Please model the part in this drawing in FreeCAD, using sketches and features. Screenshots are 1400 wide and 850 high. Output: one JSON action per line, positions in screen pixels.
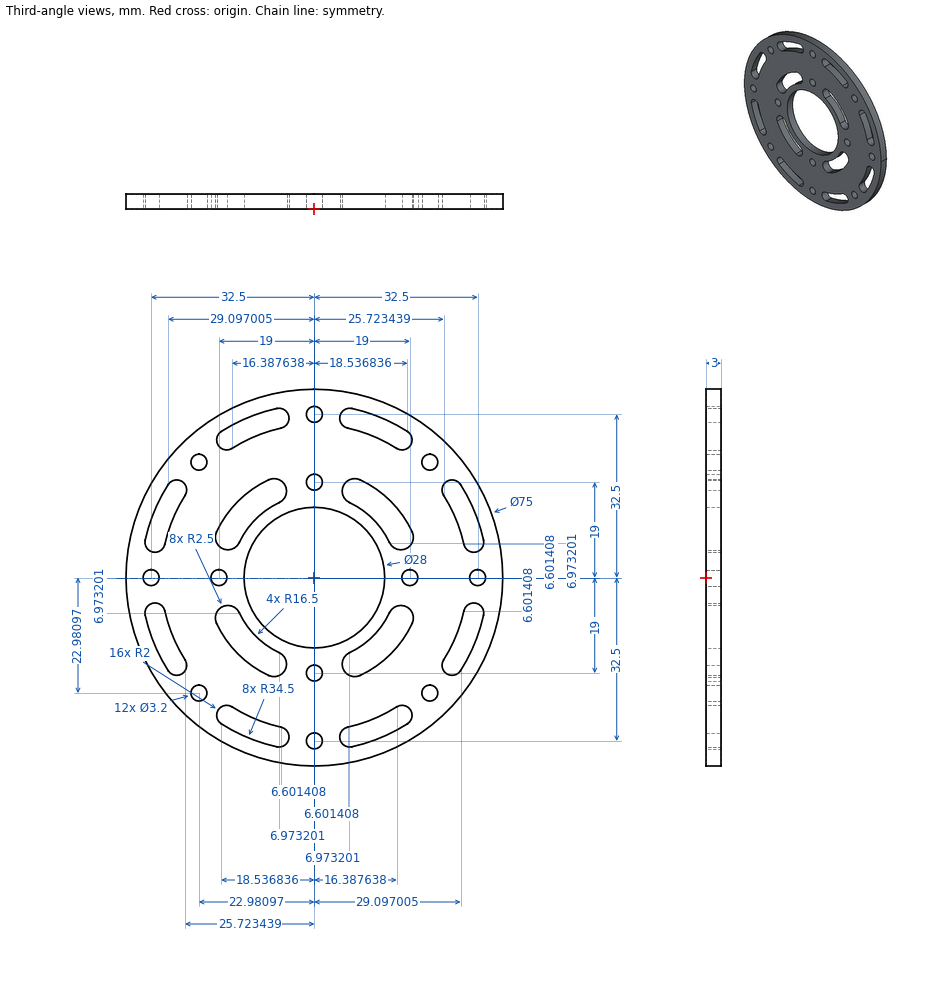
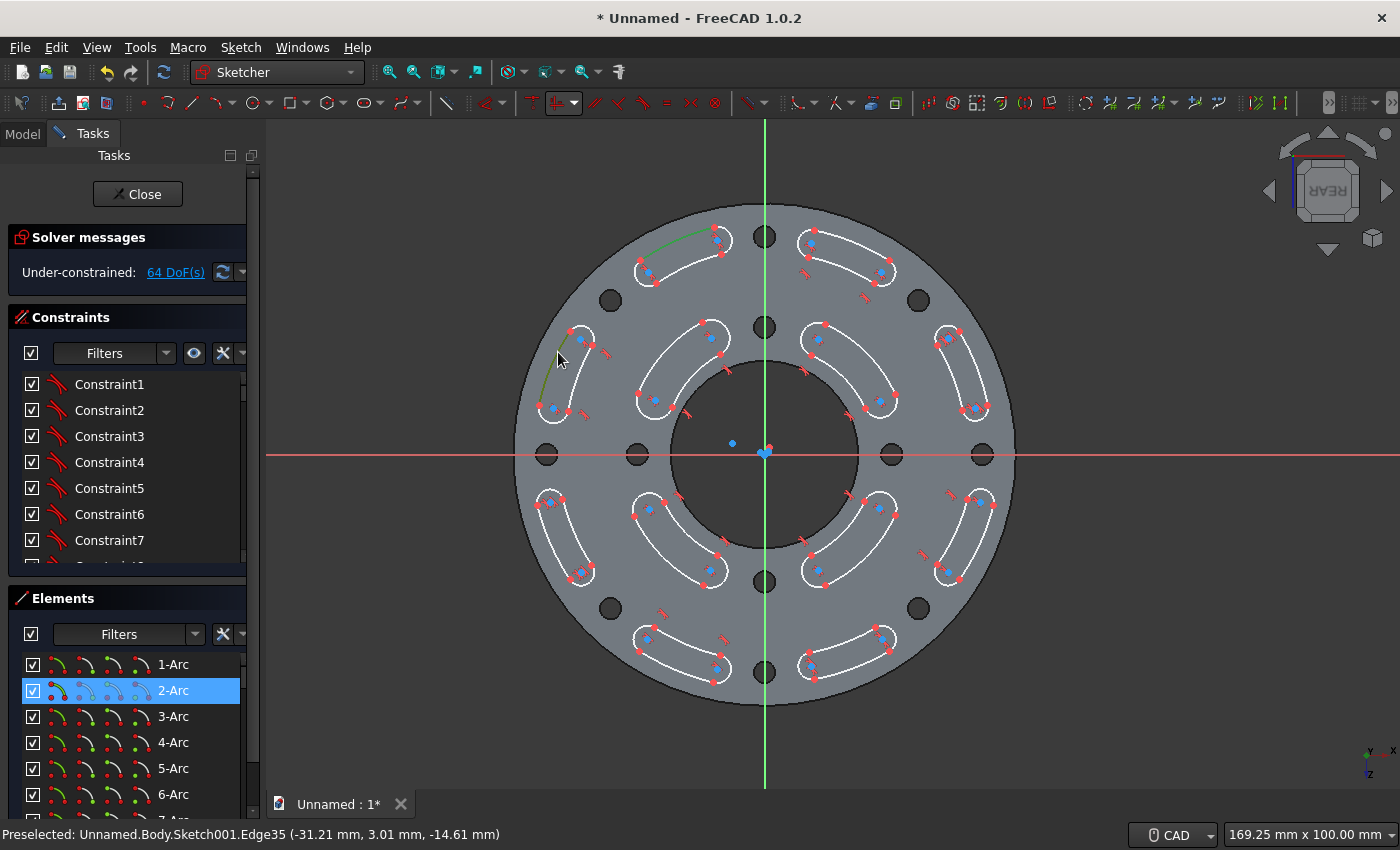
{"action": "left_click", "coordinate": [532, 104]}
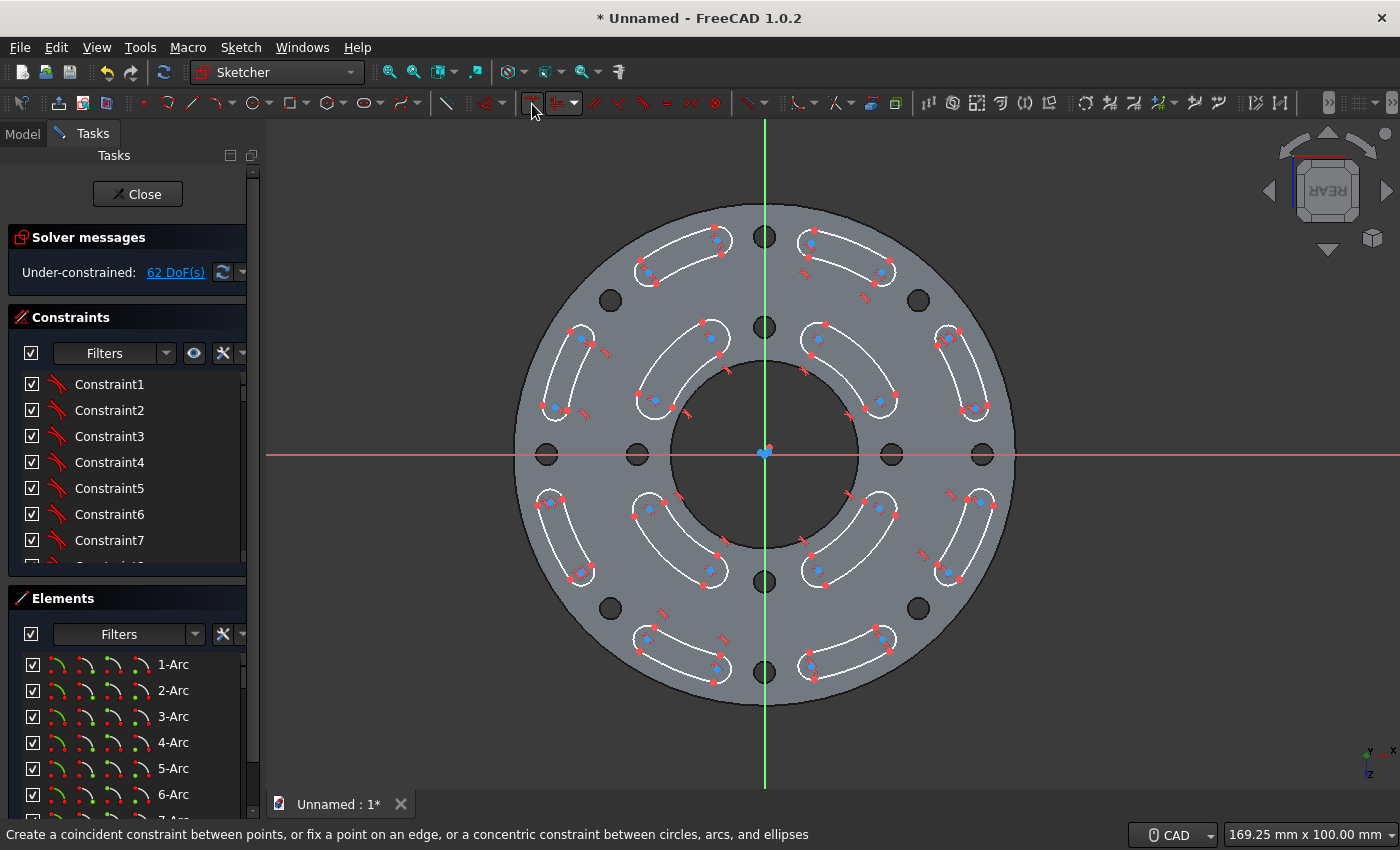
{"action": "left_click", "coordinate": [691, 234]}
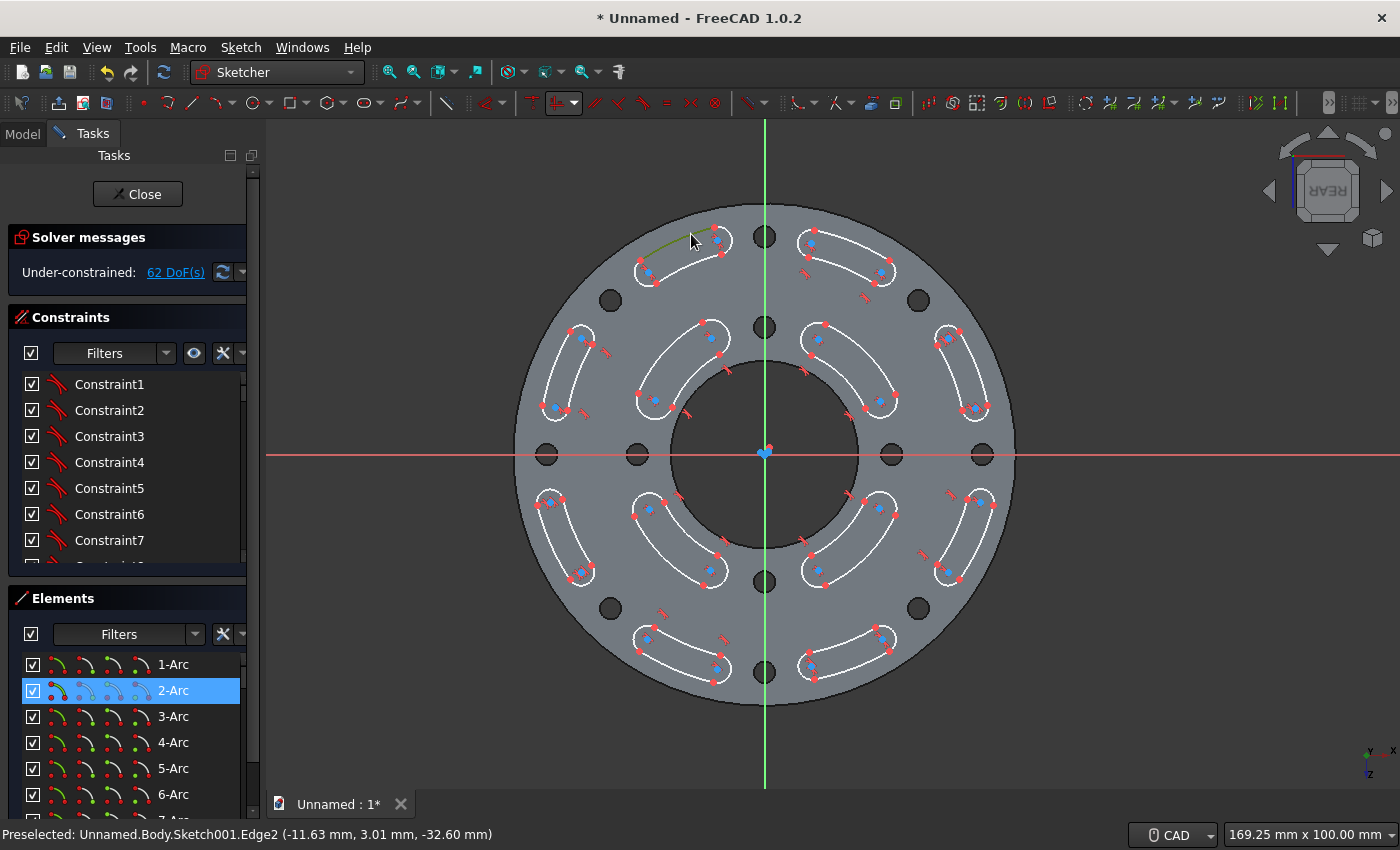
{"action": "left_click", "coordinate": [853, 388]}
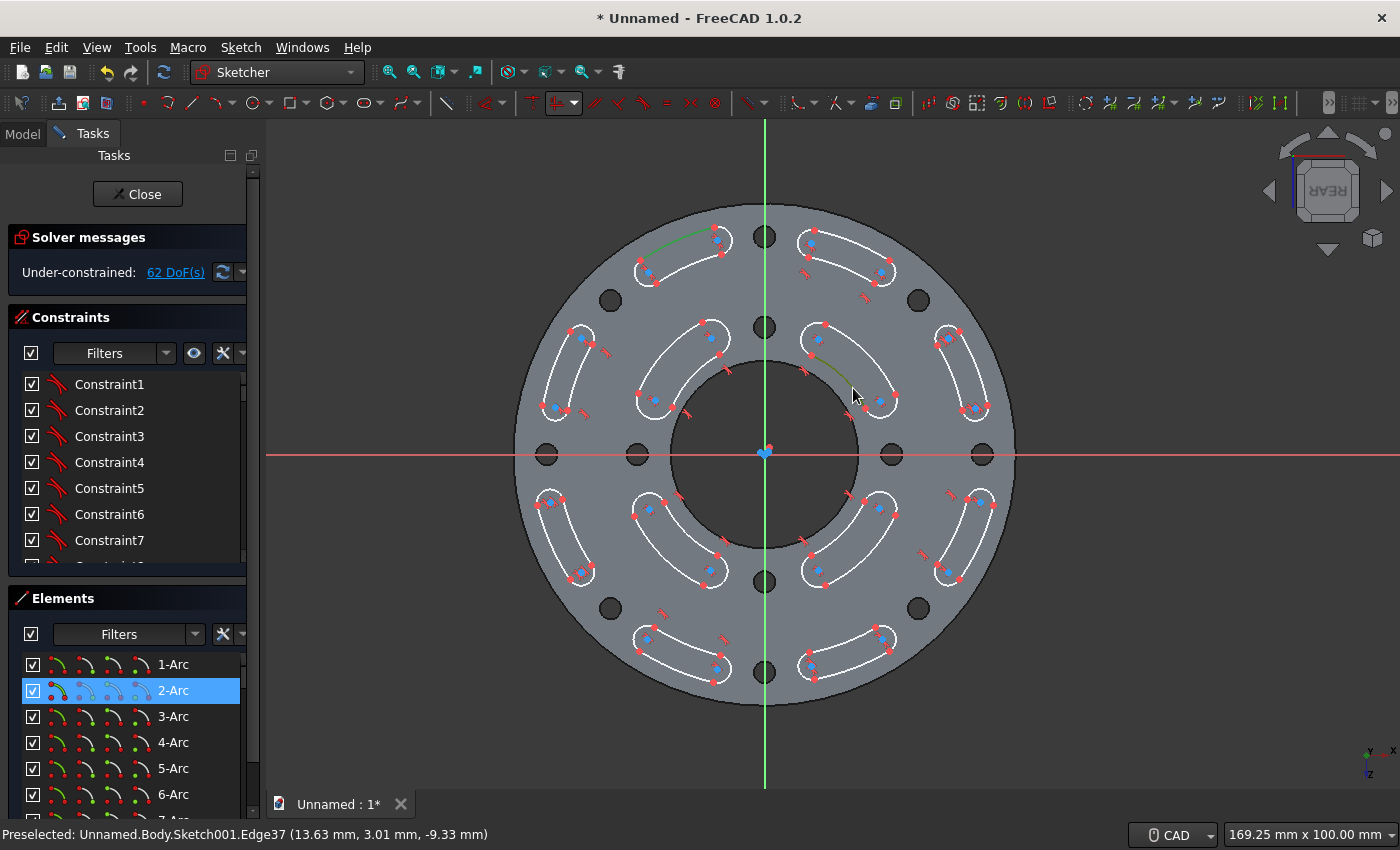
{"action": "left_click", "coordinate": [532, 104]}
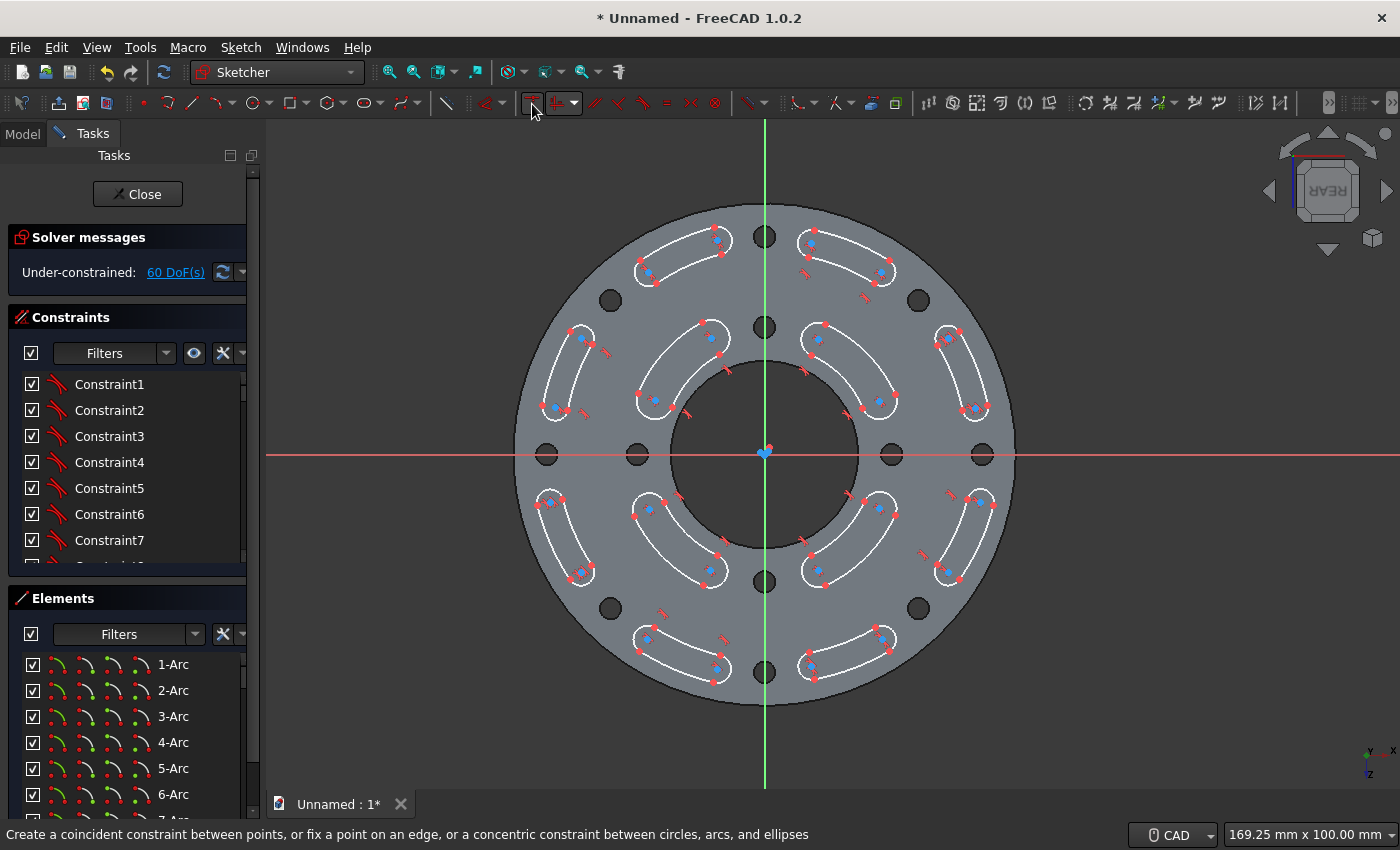
{"action": "left_click", "coordinate": [691, 235]}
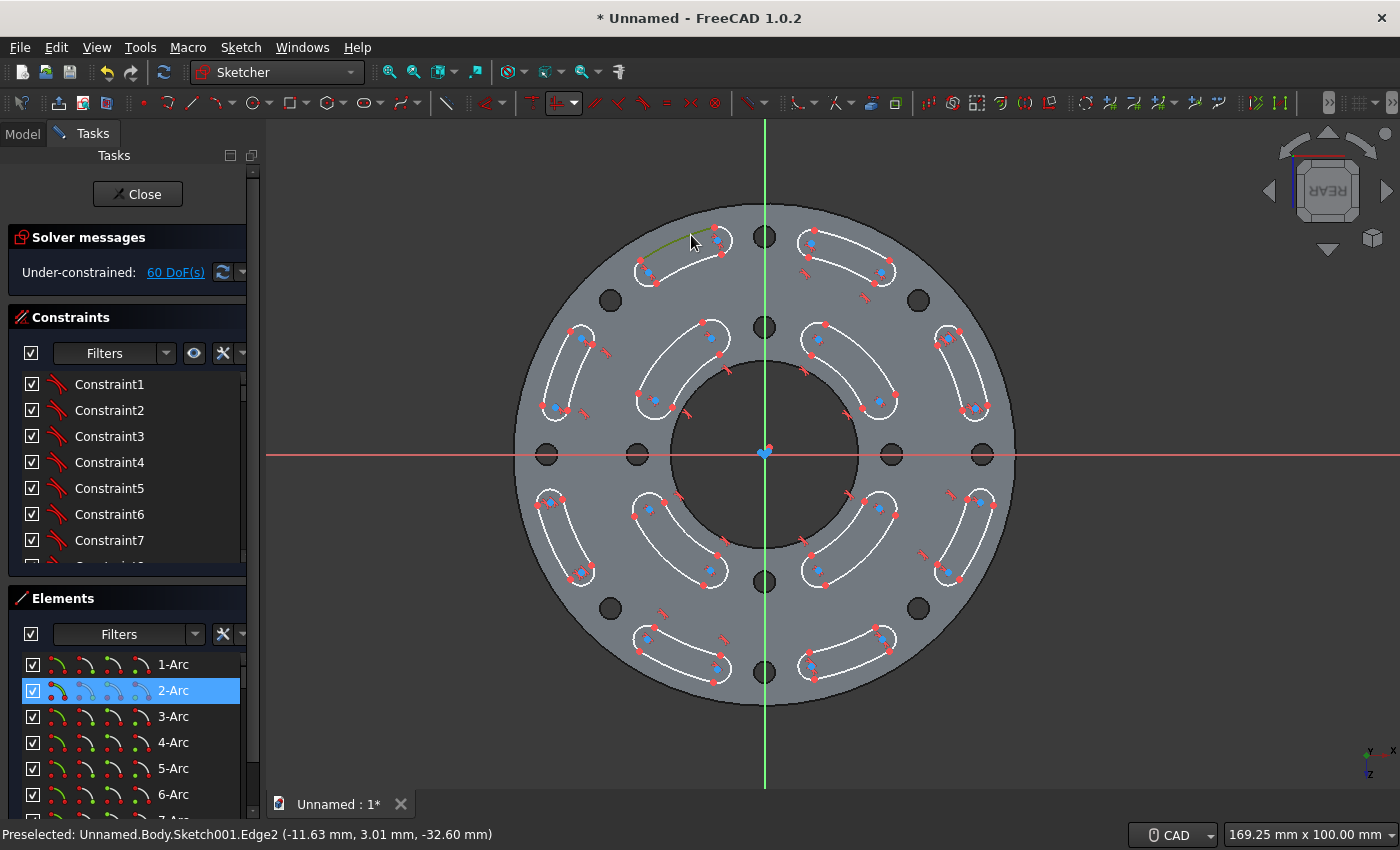
{"action": "left_click", "coordinate": [880, 368]}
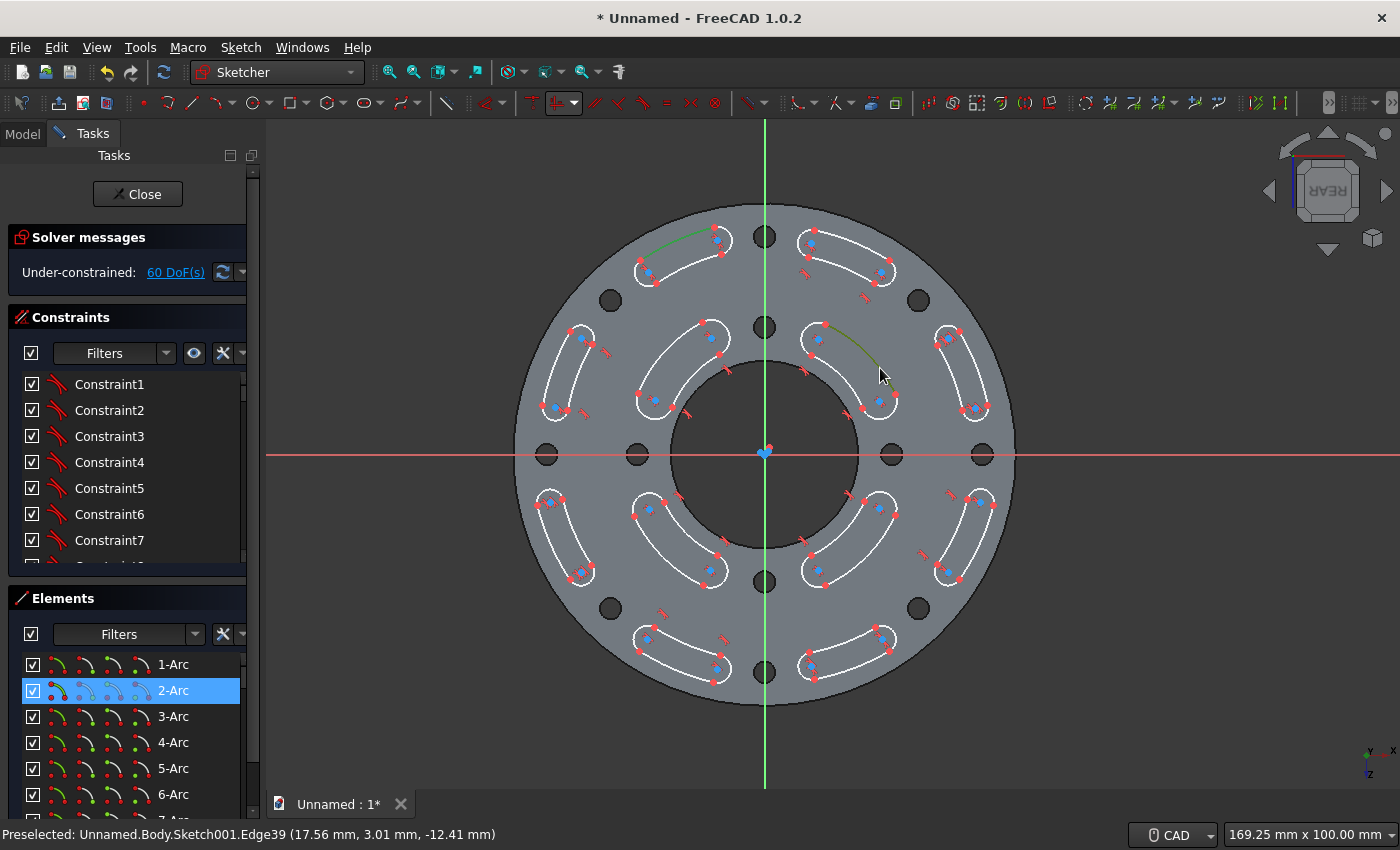
{"action": "left_click", "coordinate": [532, 104]}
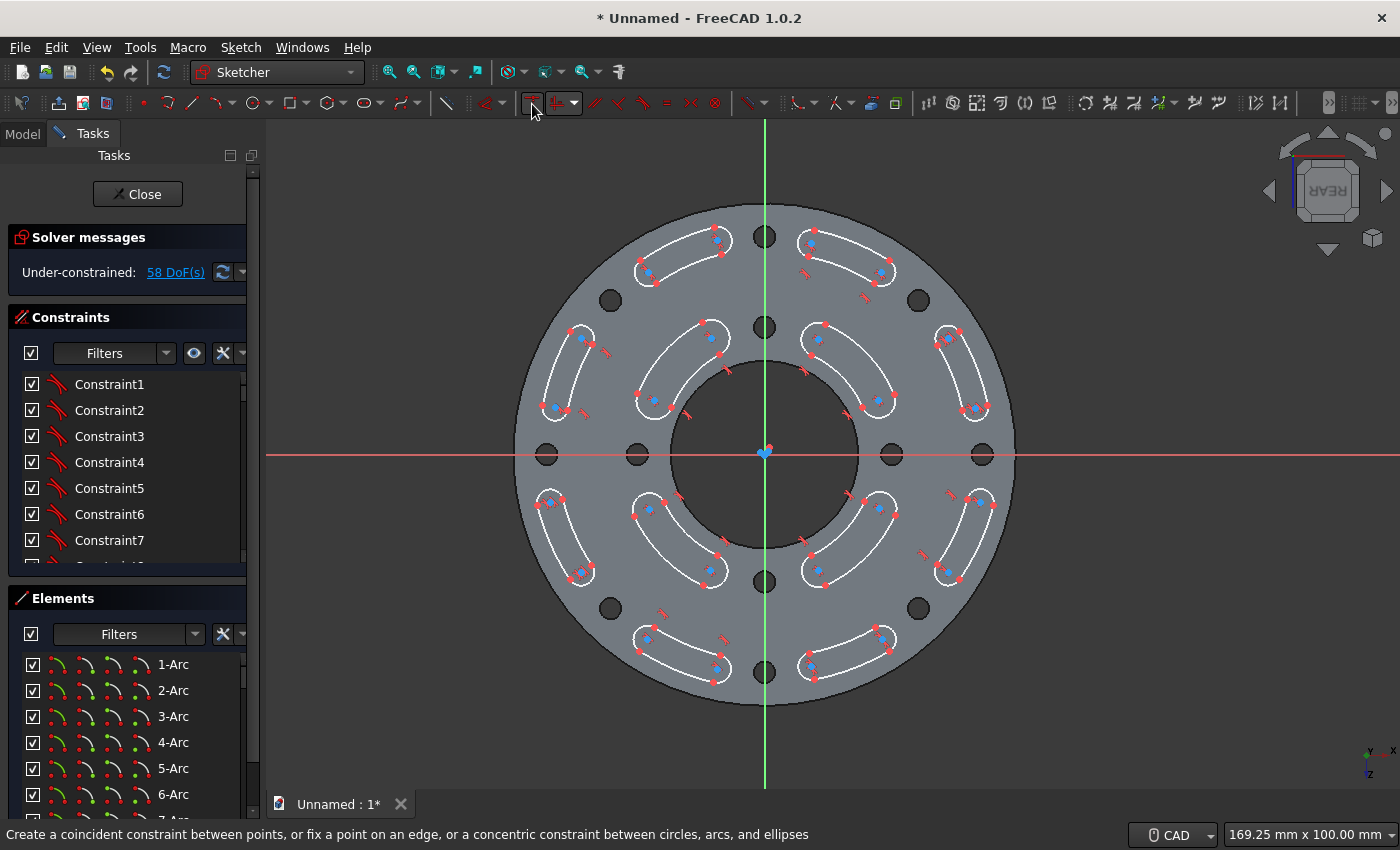
{"action": "left_click", "coordinate": [691, 235]}